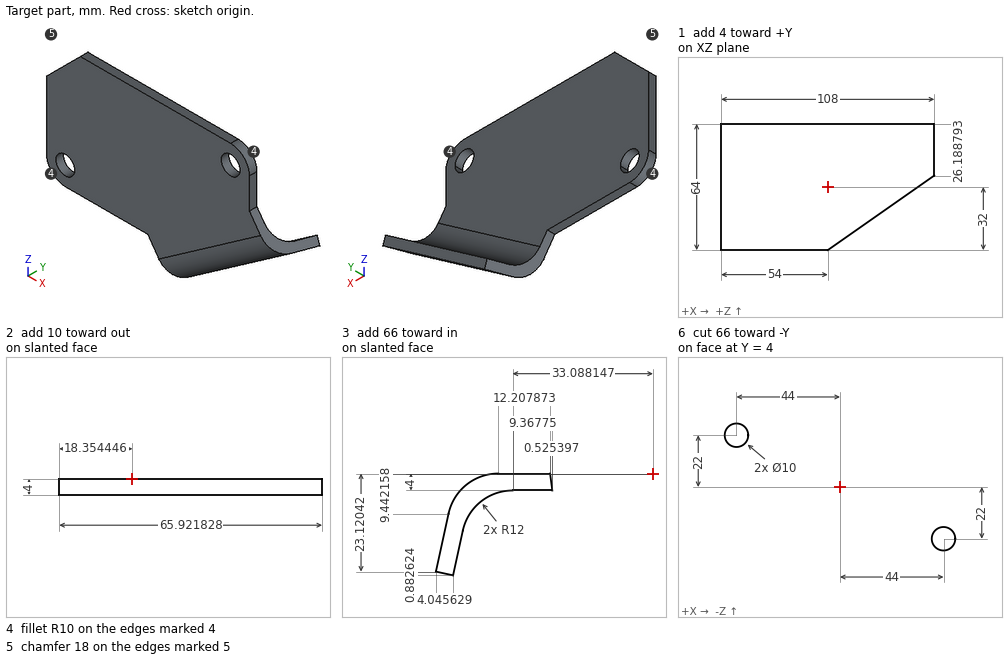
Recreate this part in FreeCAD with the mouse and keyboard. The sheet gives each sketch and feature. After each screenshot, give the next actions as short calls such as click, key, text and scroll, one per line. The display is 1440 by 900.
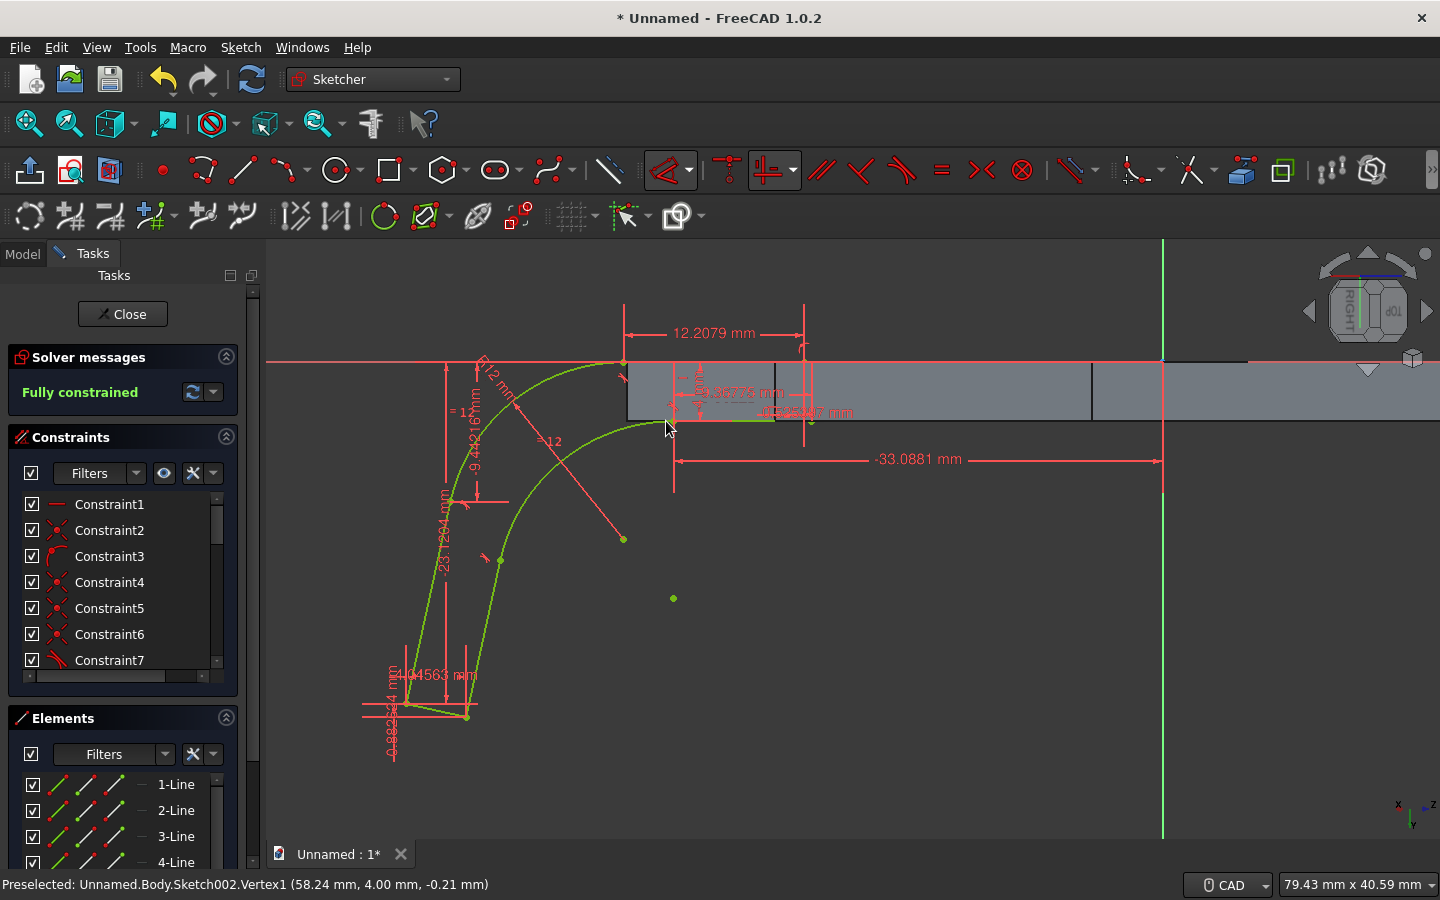
click(123, 314)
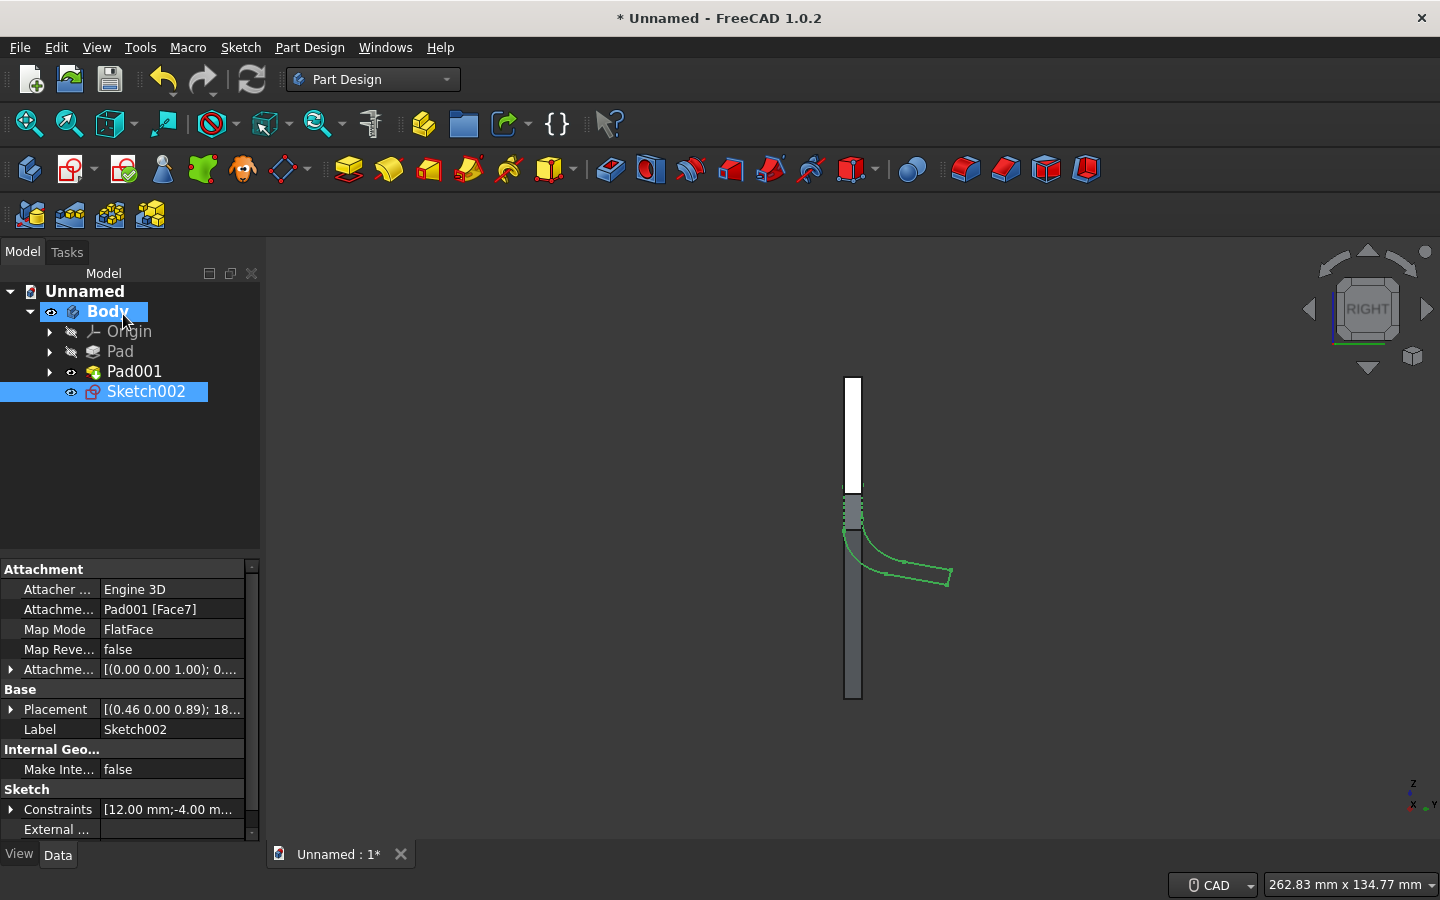
click(350, 170)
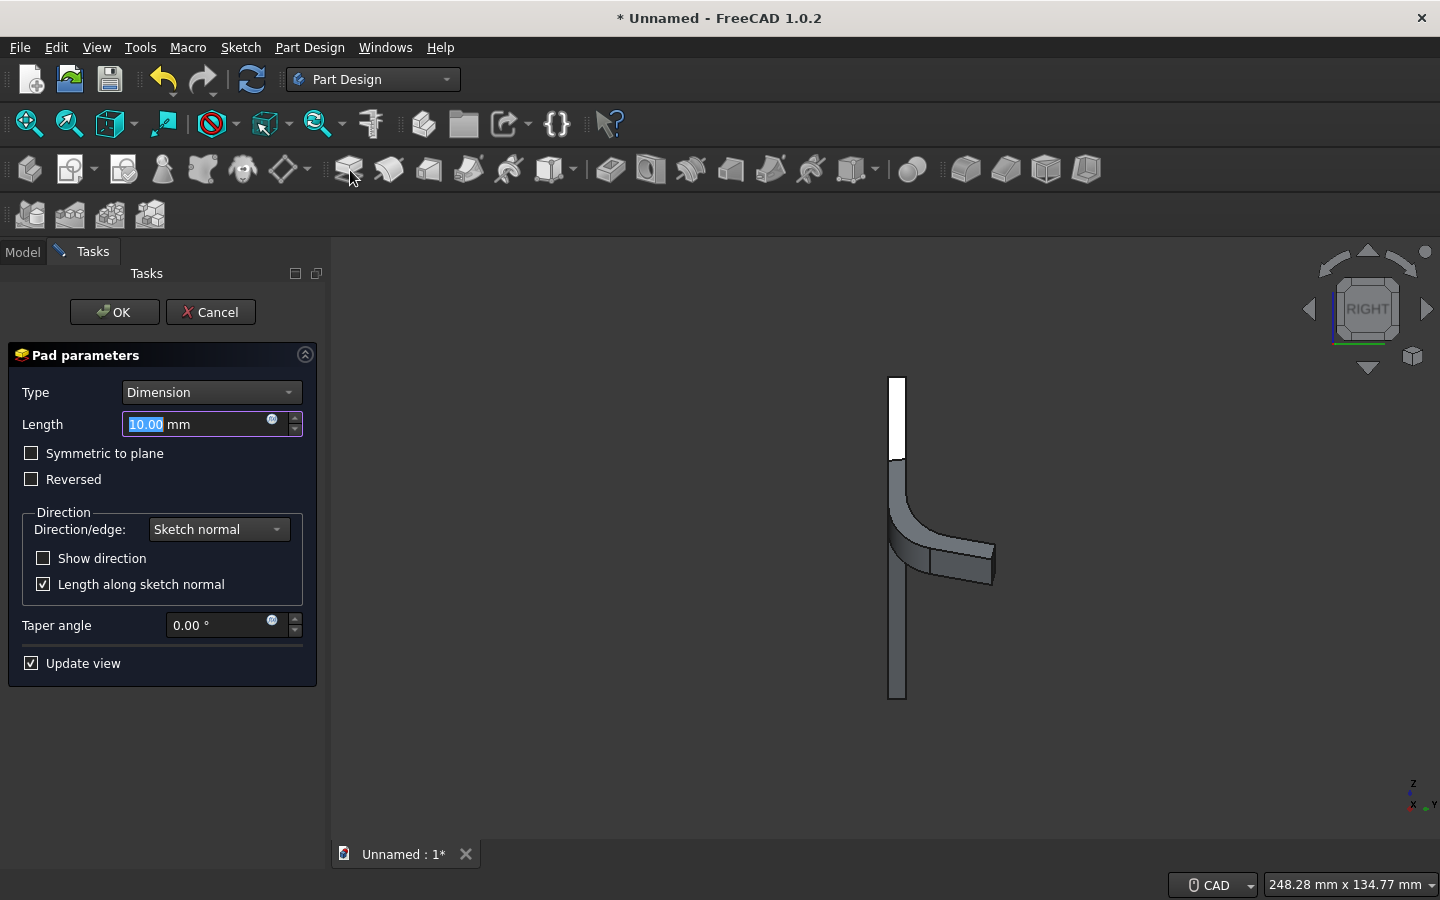
text(66)
key(Tab)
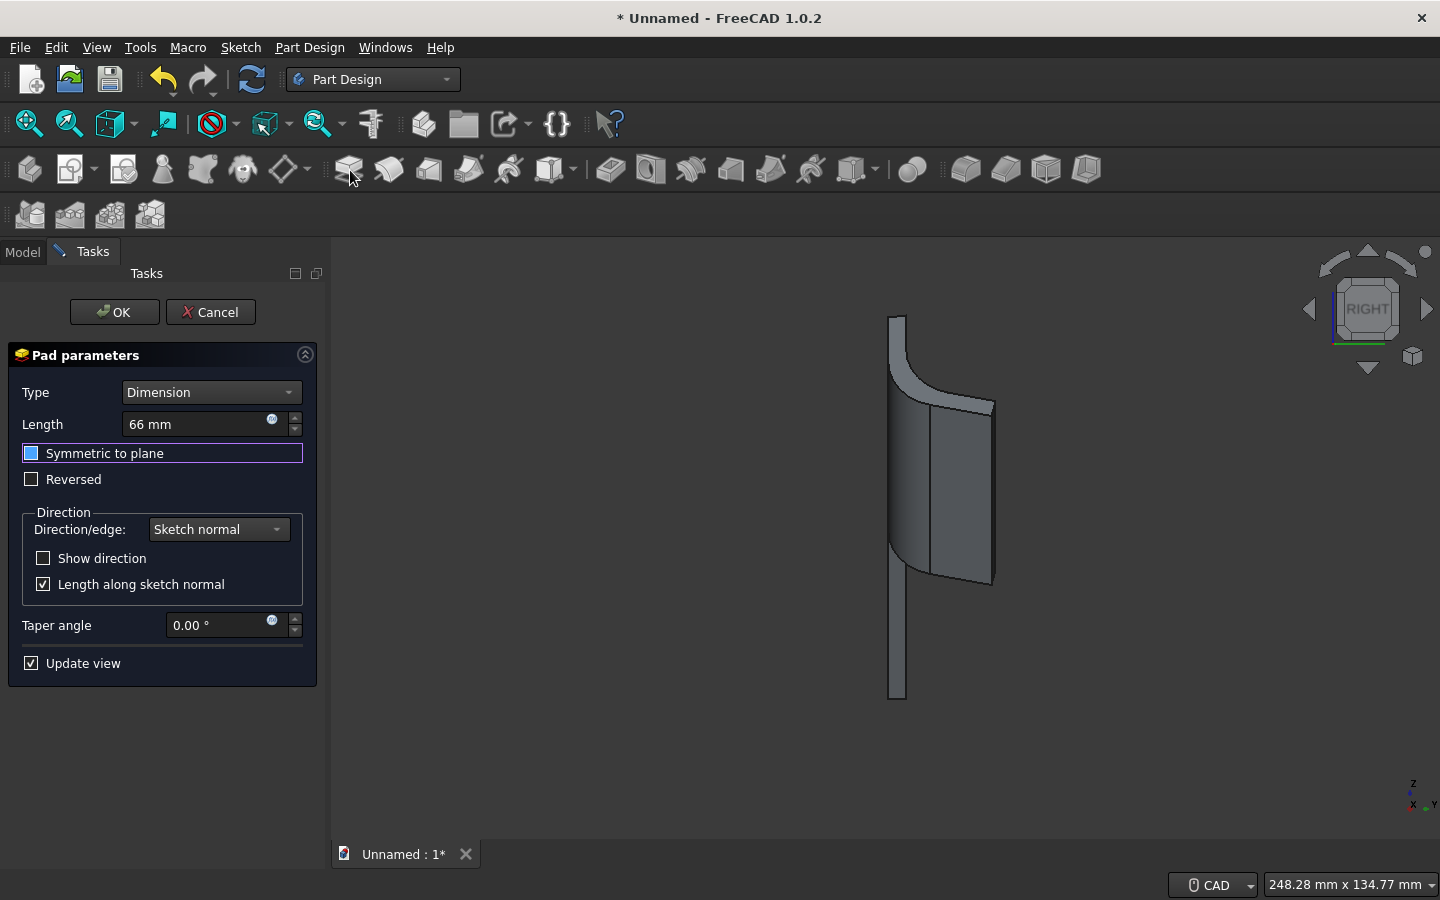
click(30, 479)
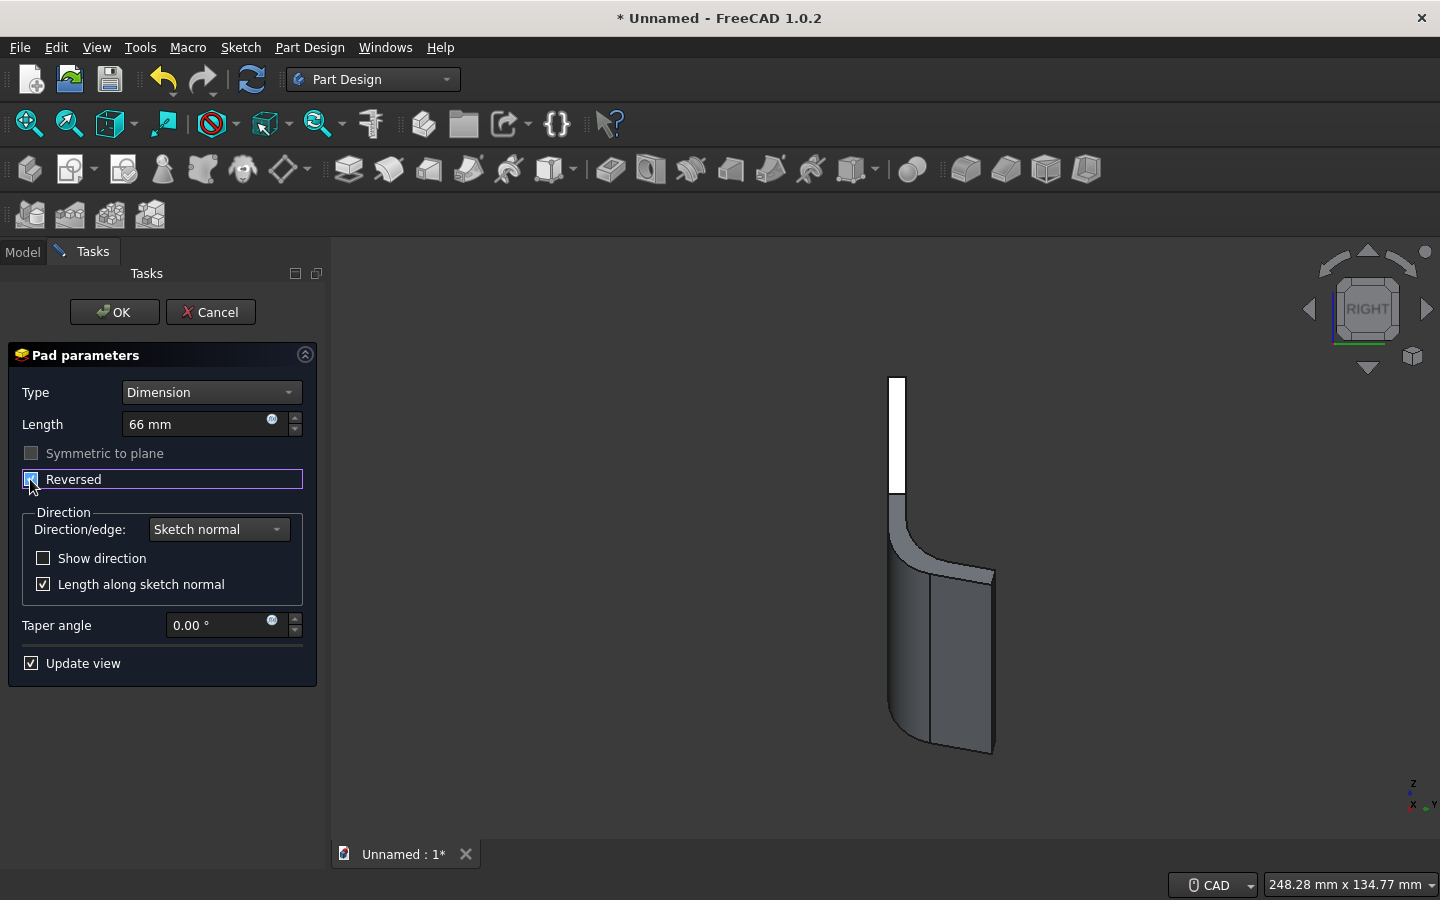
click(115, 312)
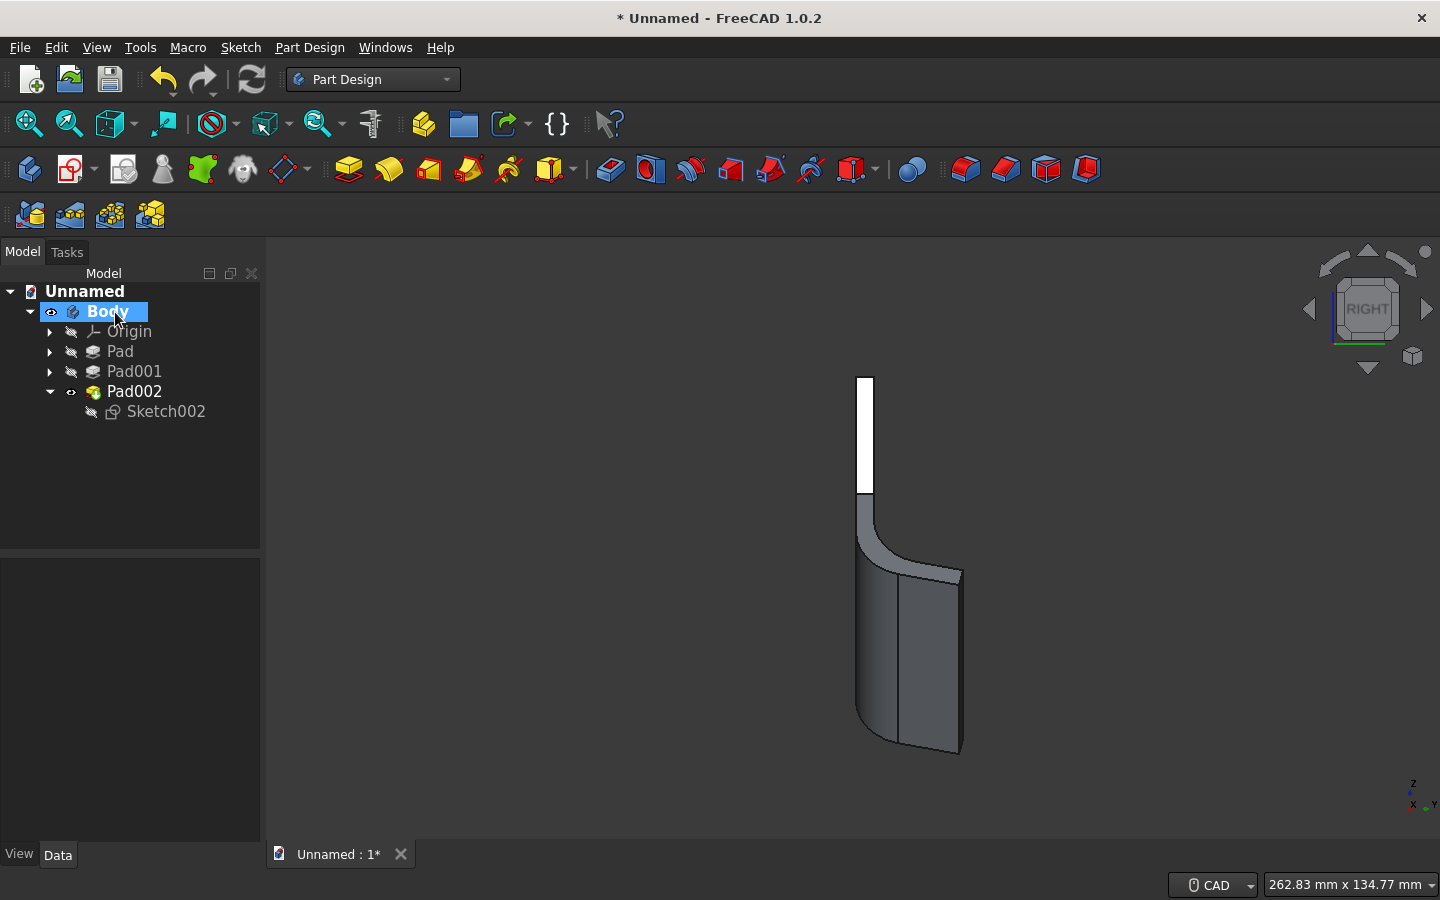
scroll(865, 662, up, 5)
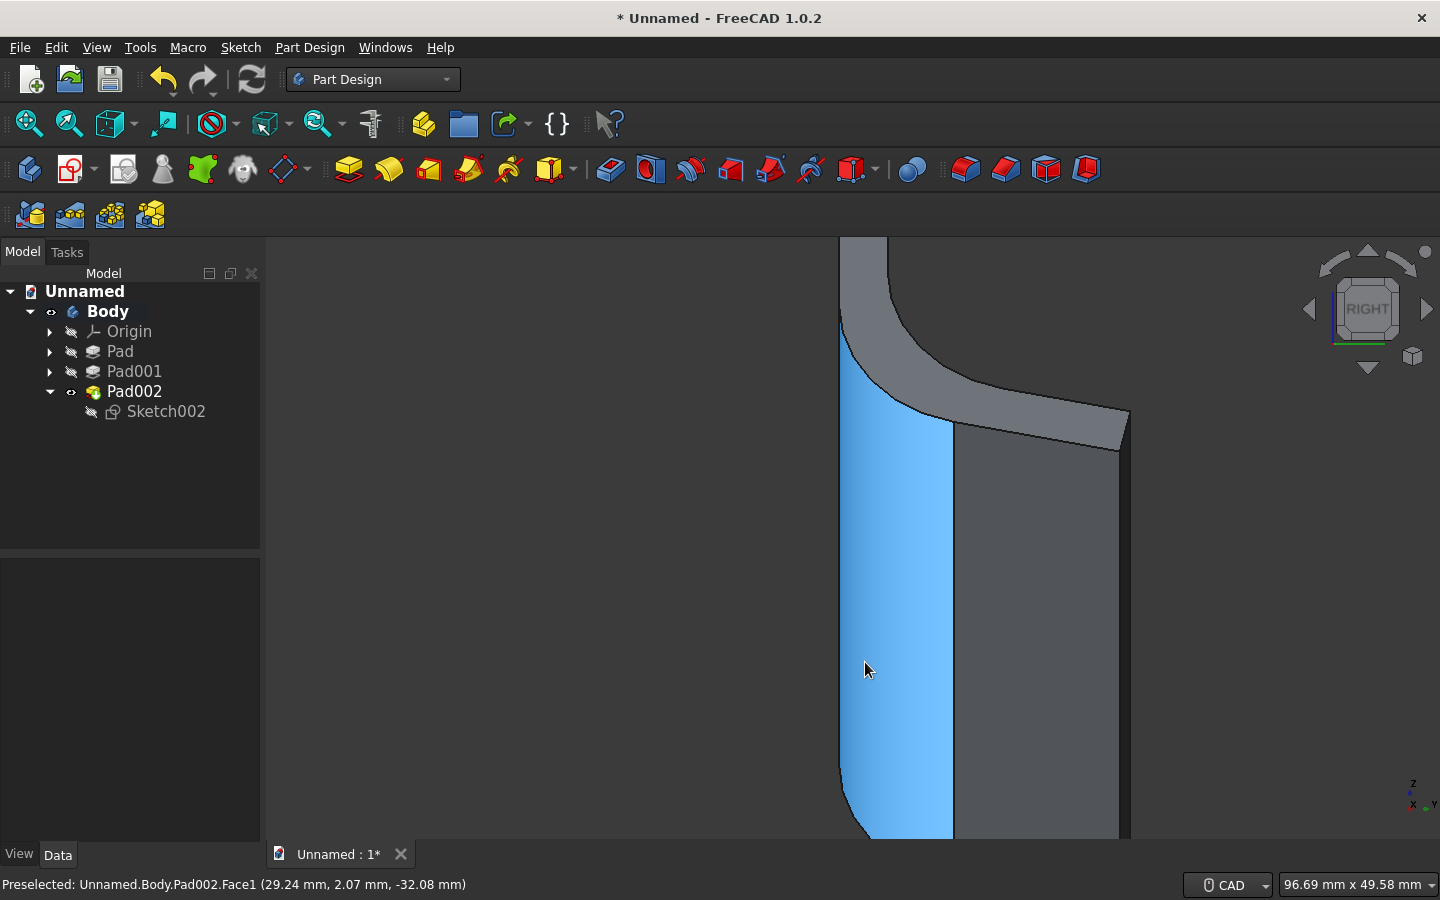
key(v)
key(f)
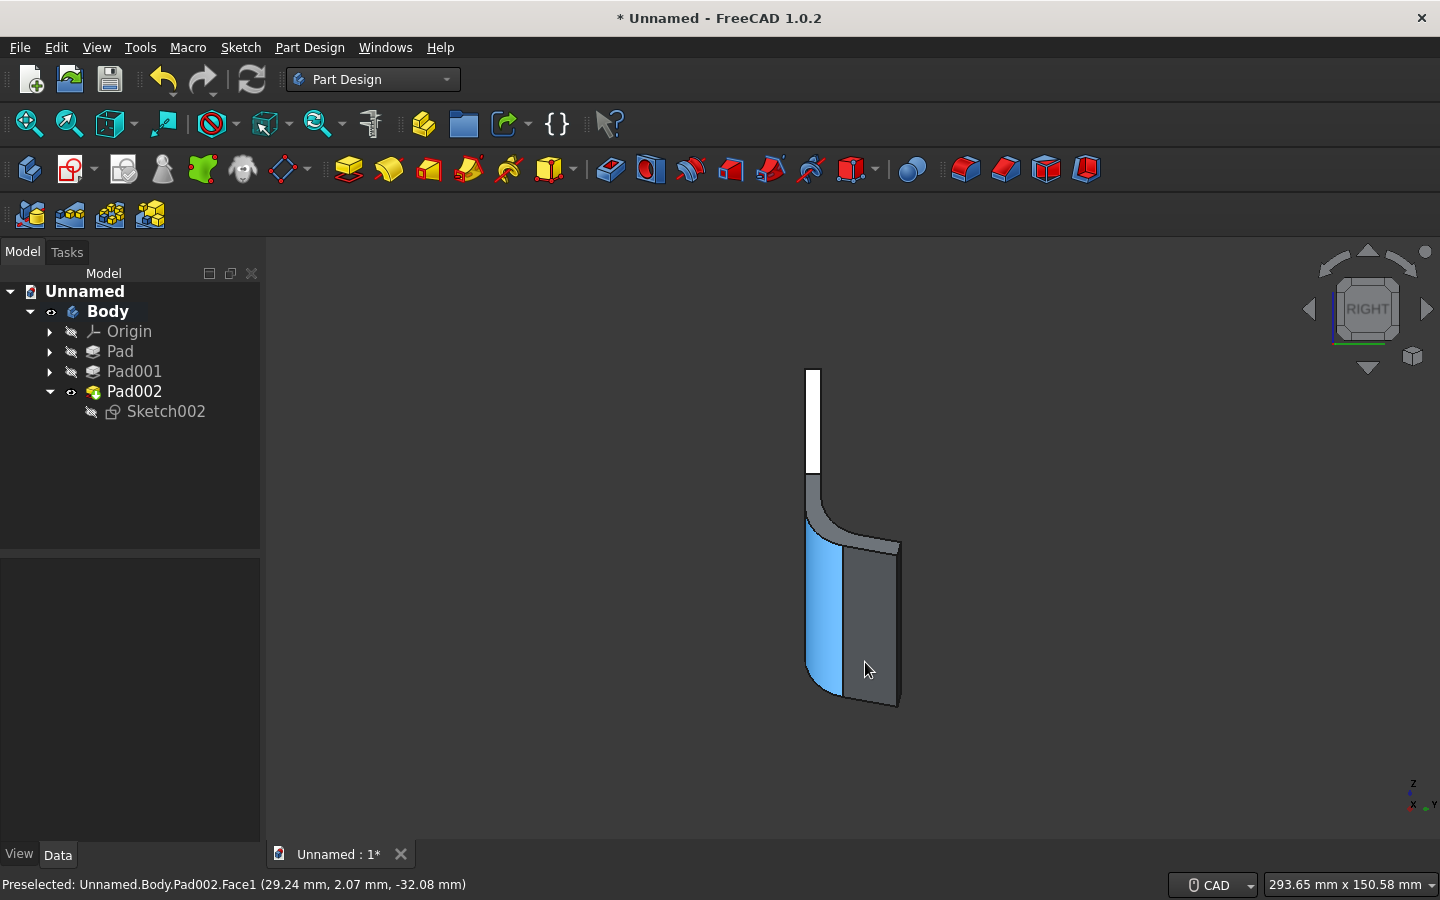
key(0)